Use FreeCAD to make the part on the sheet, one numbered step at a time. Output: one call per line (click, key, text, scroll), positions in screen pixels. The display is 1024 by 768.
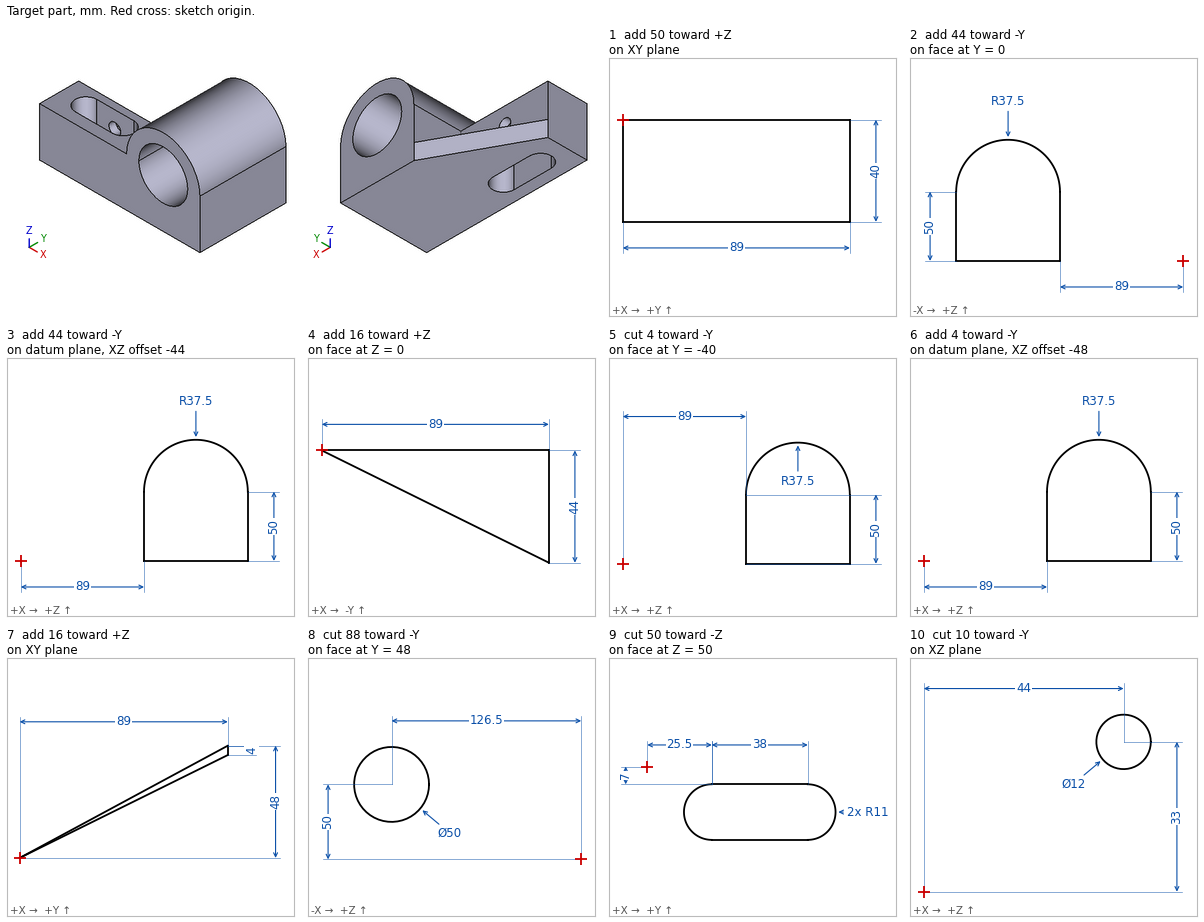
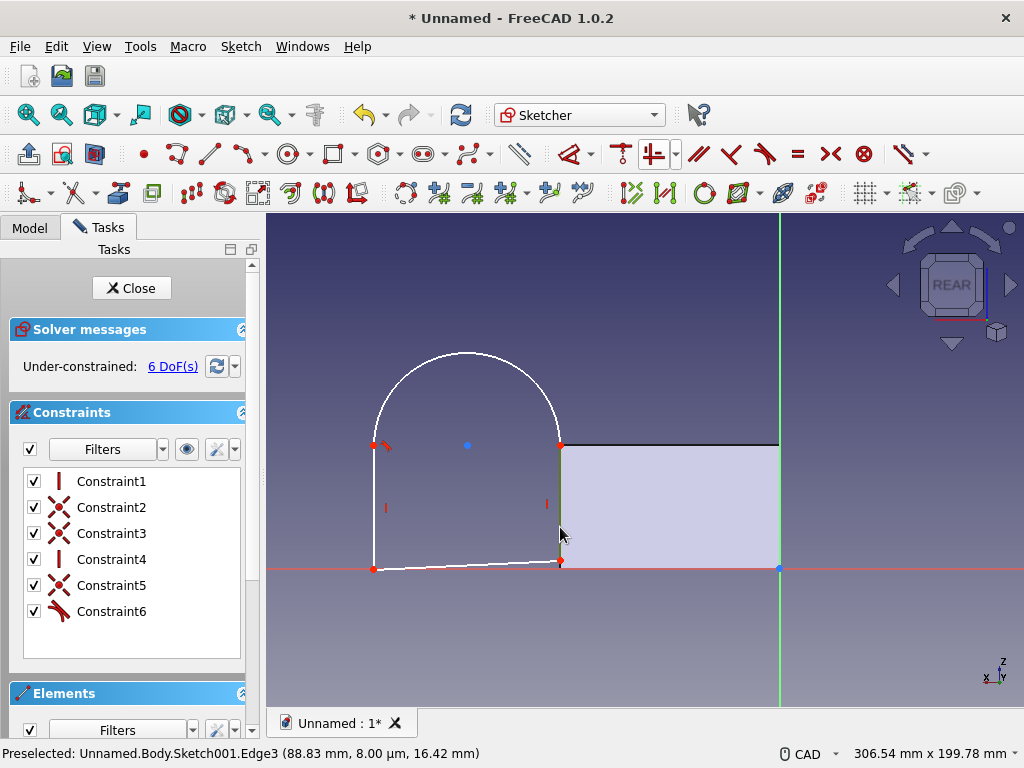
click(522, 371)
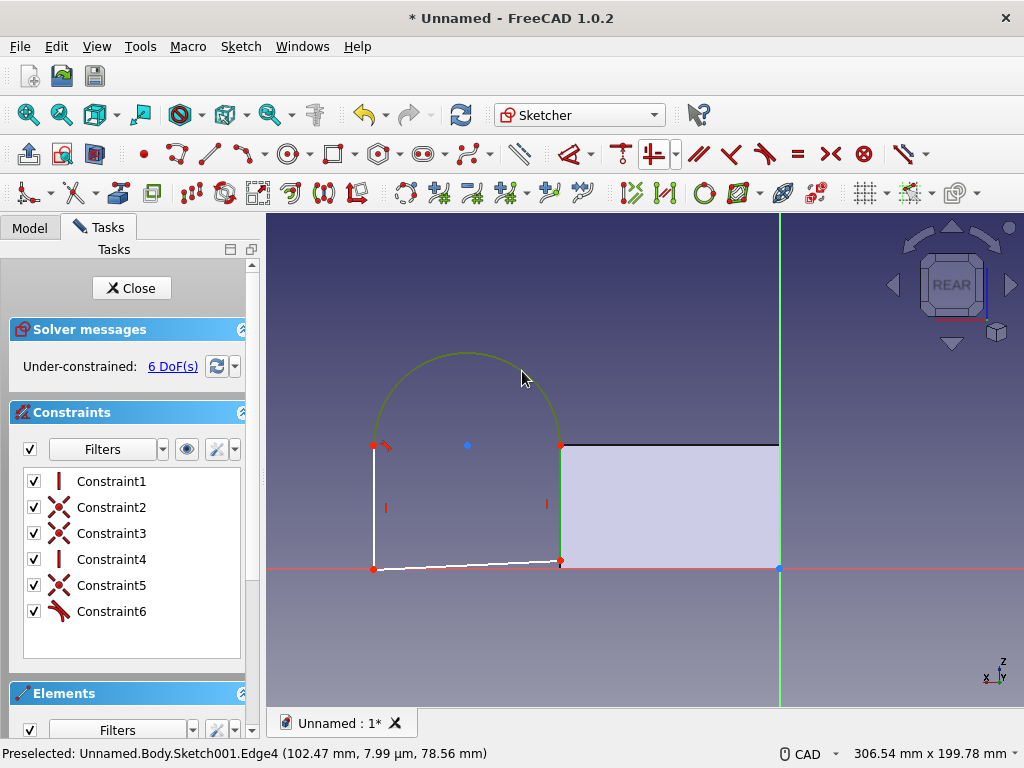
click(765, 154)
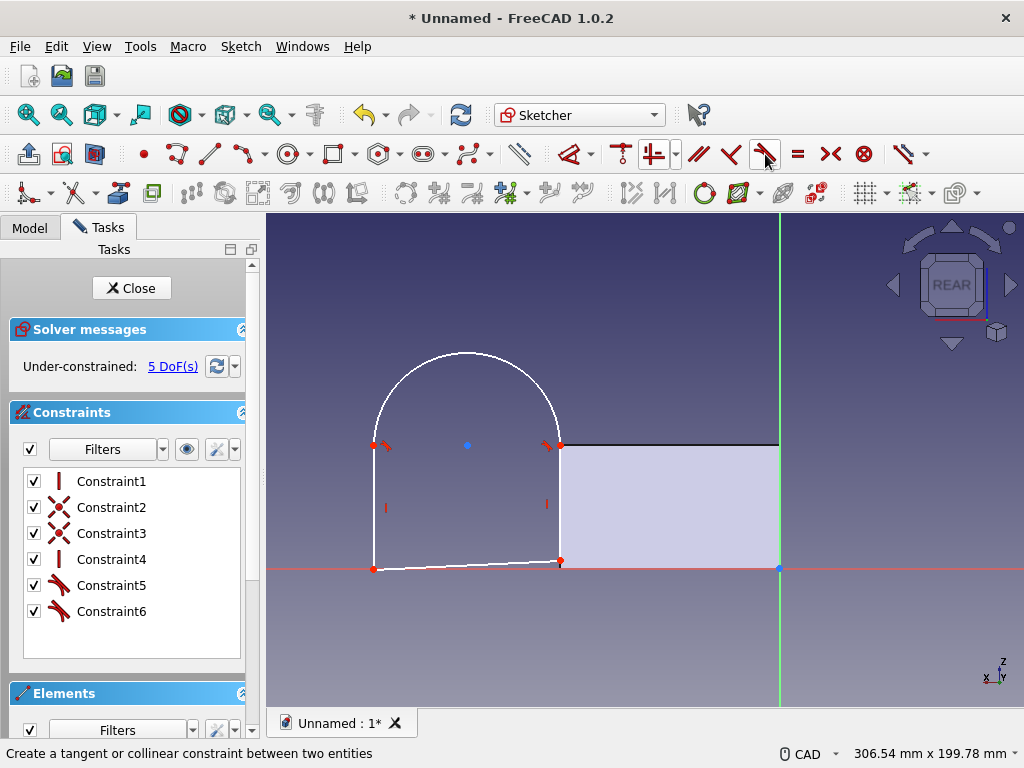
click(430, 567)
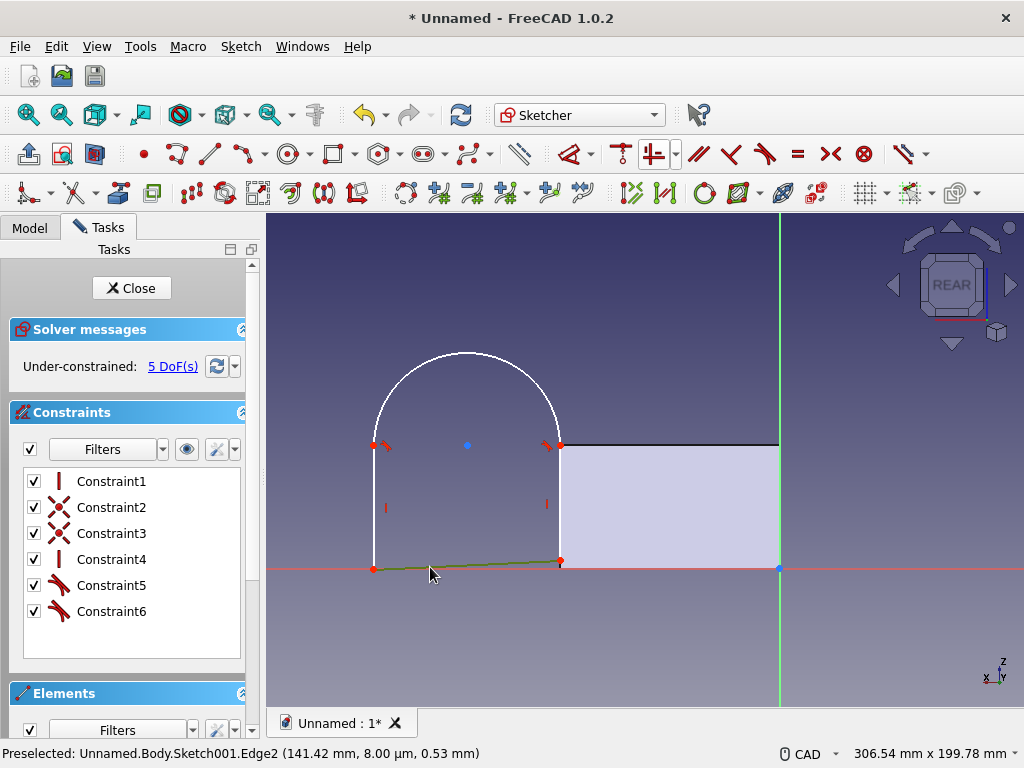
key(h)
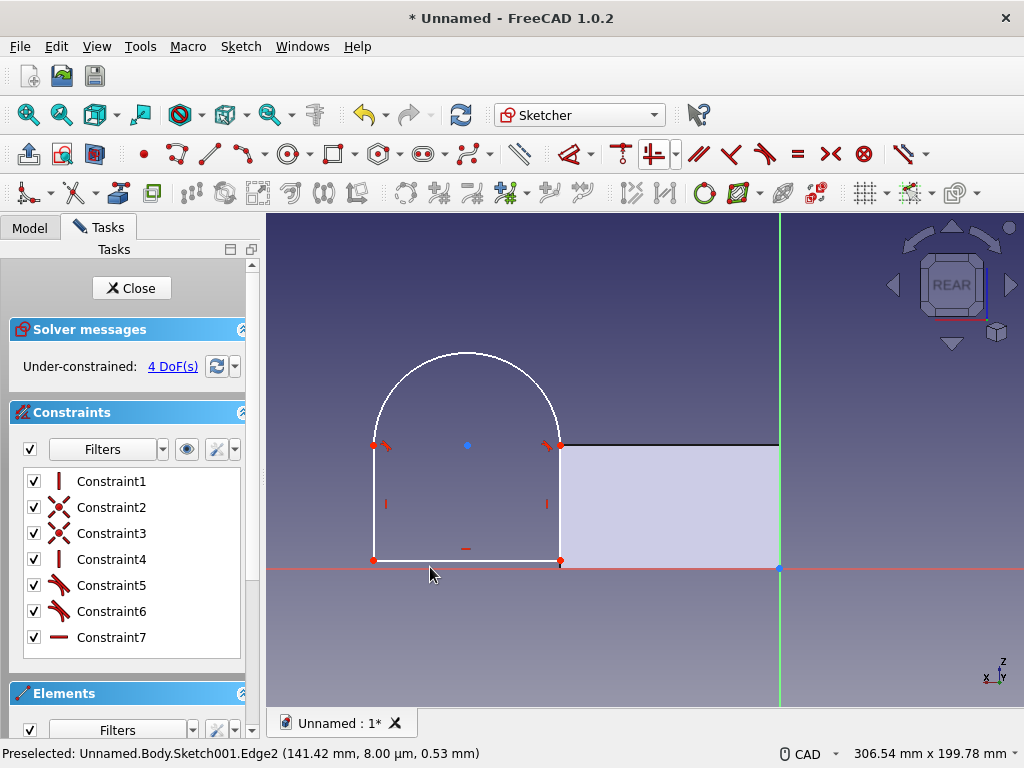
key(d)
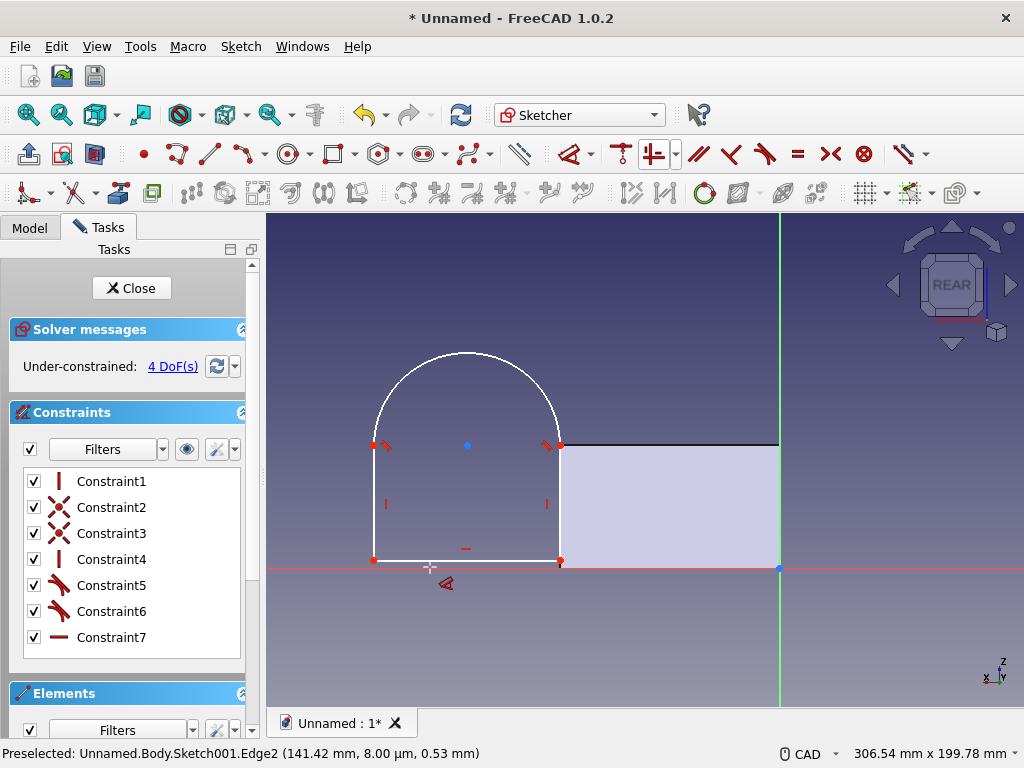
click(522, 371)
click(541, 345)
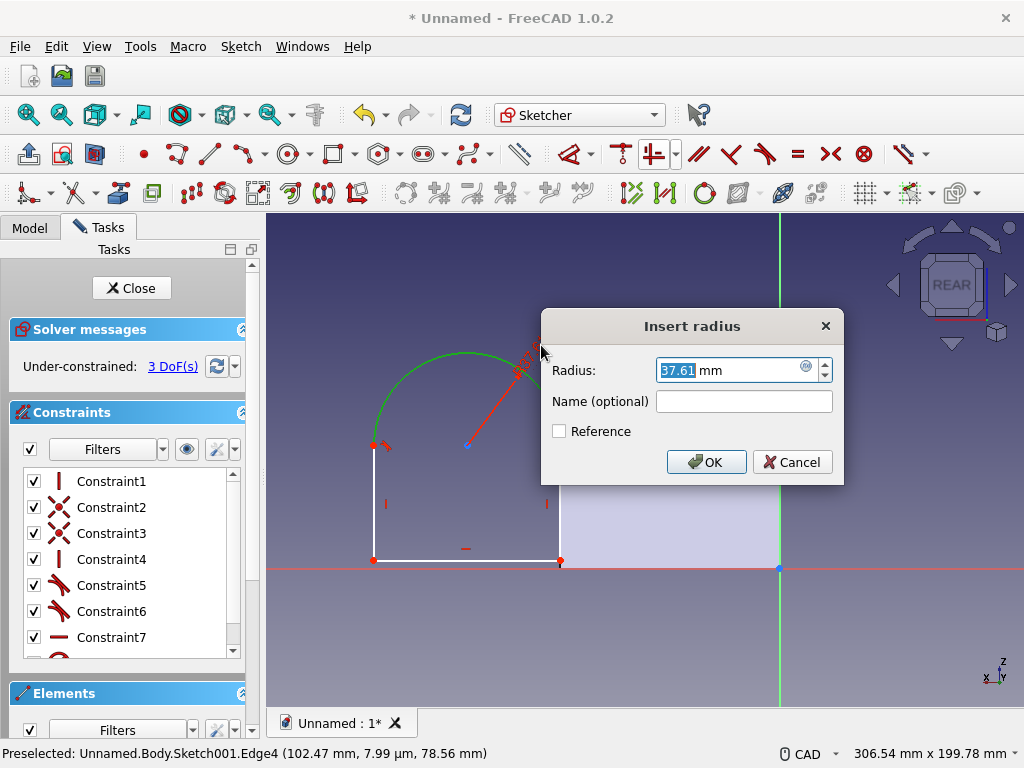
text(37.5)
key(Return)
key(Escape)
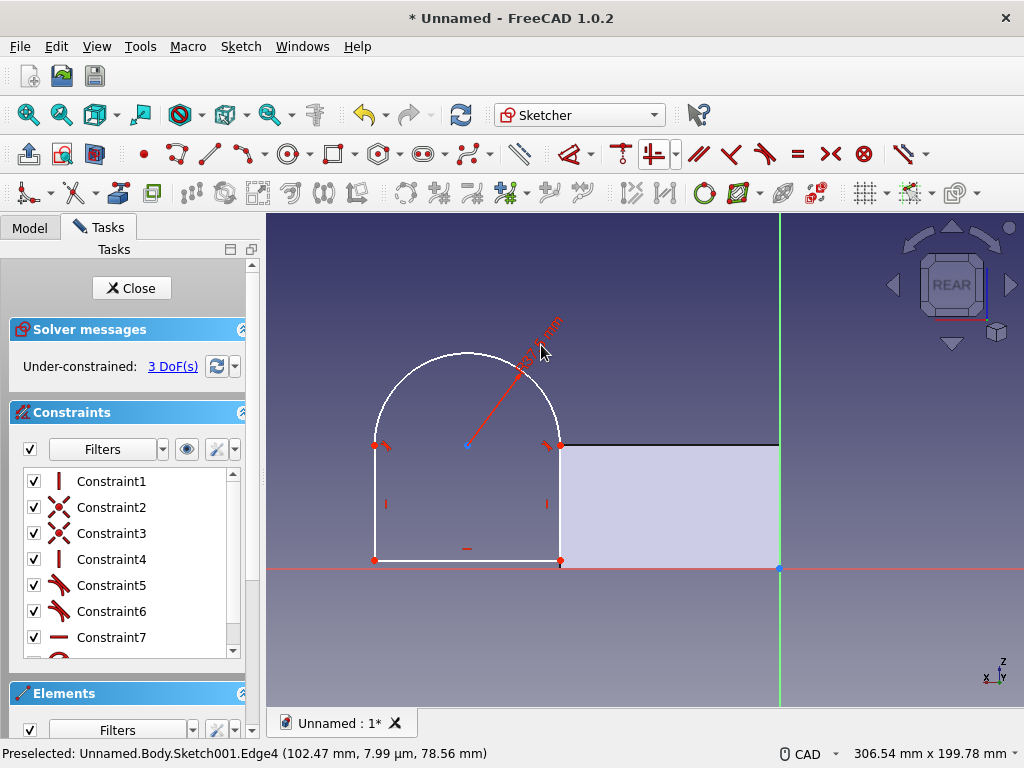
click(375, 561)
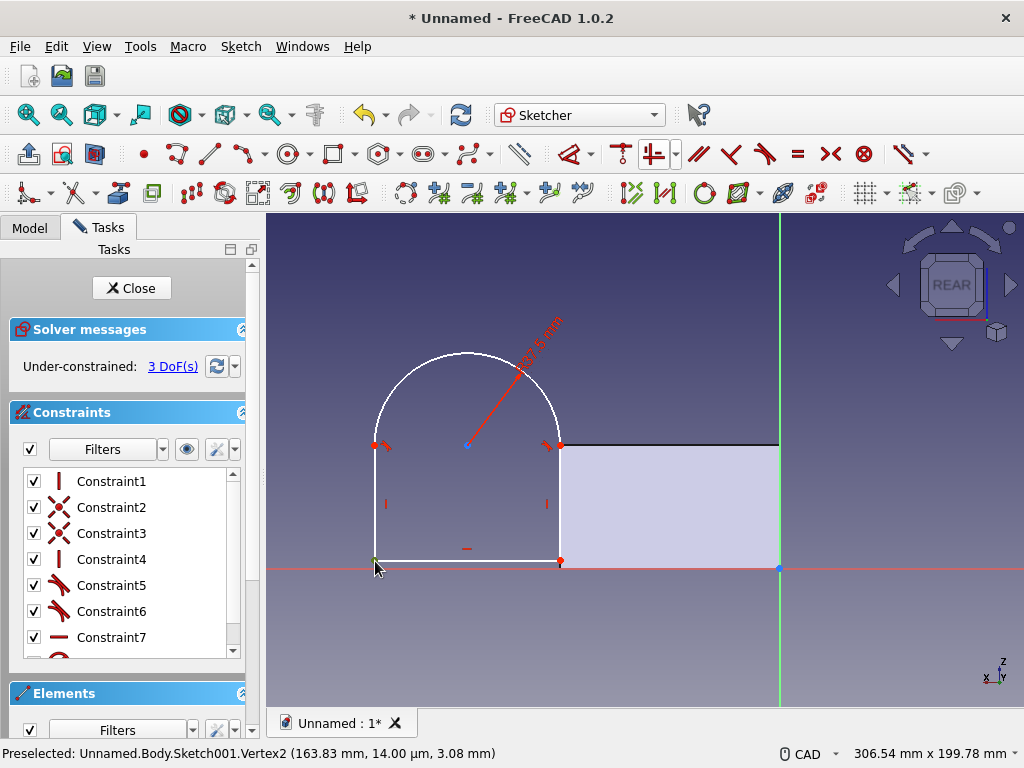
click(334, 569)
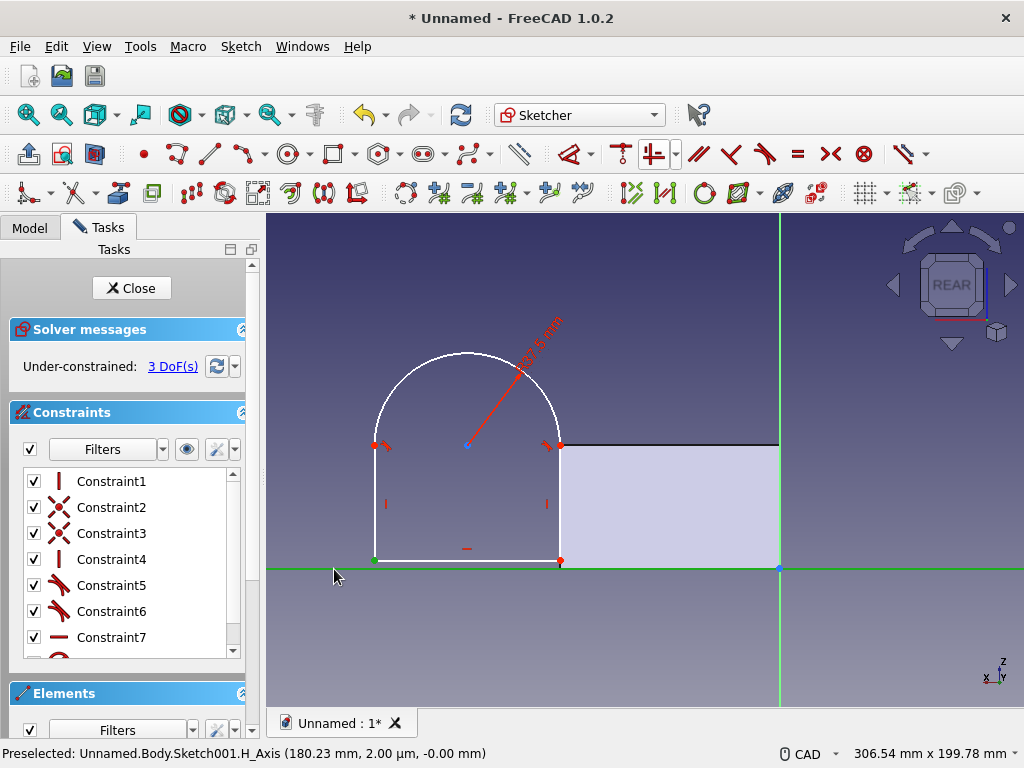
click(621, 154)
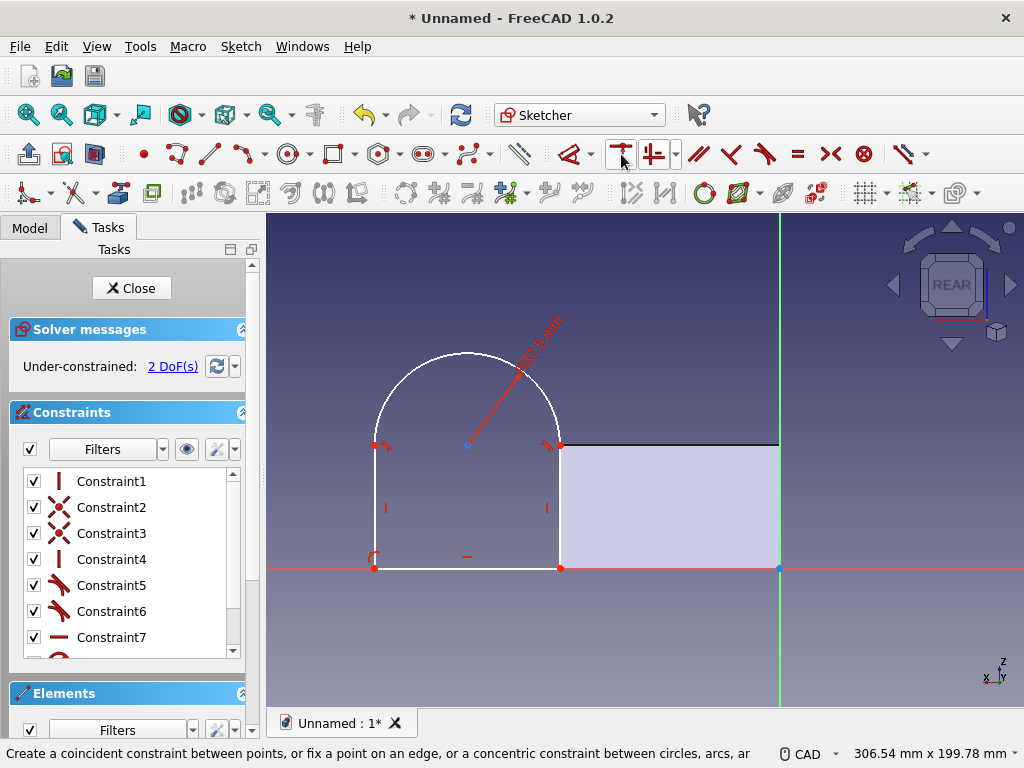
click(568, 154)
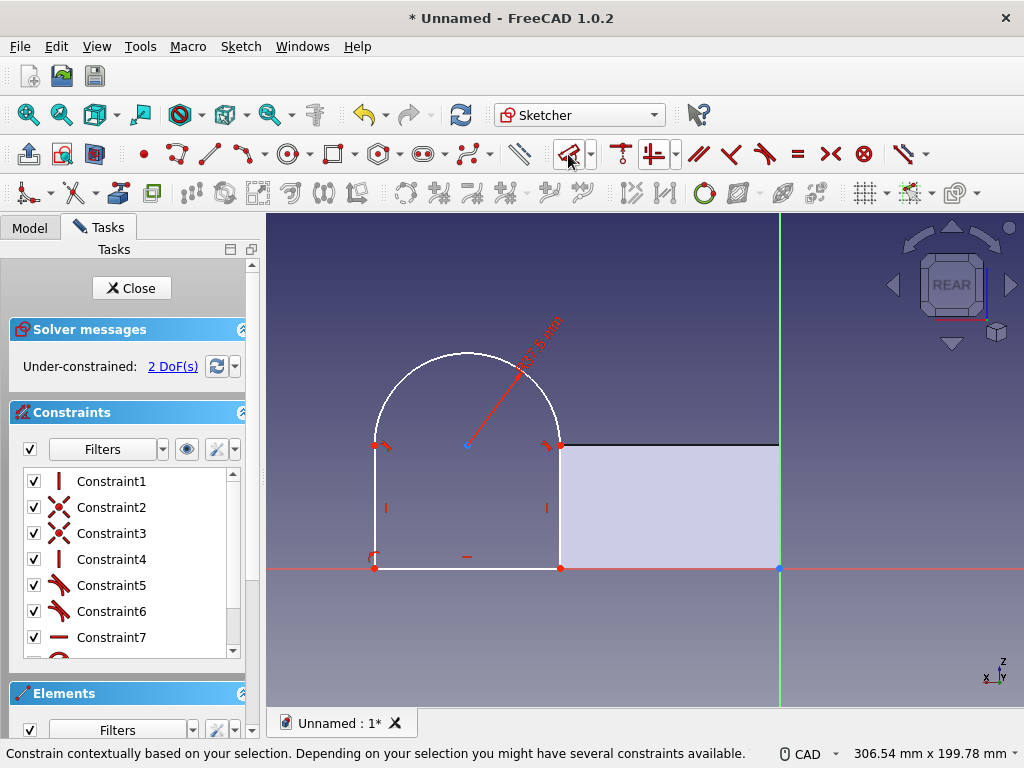
click(375, 483)
click(341, 507)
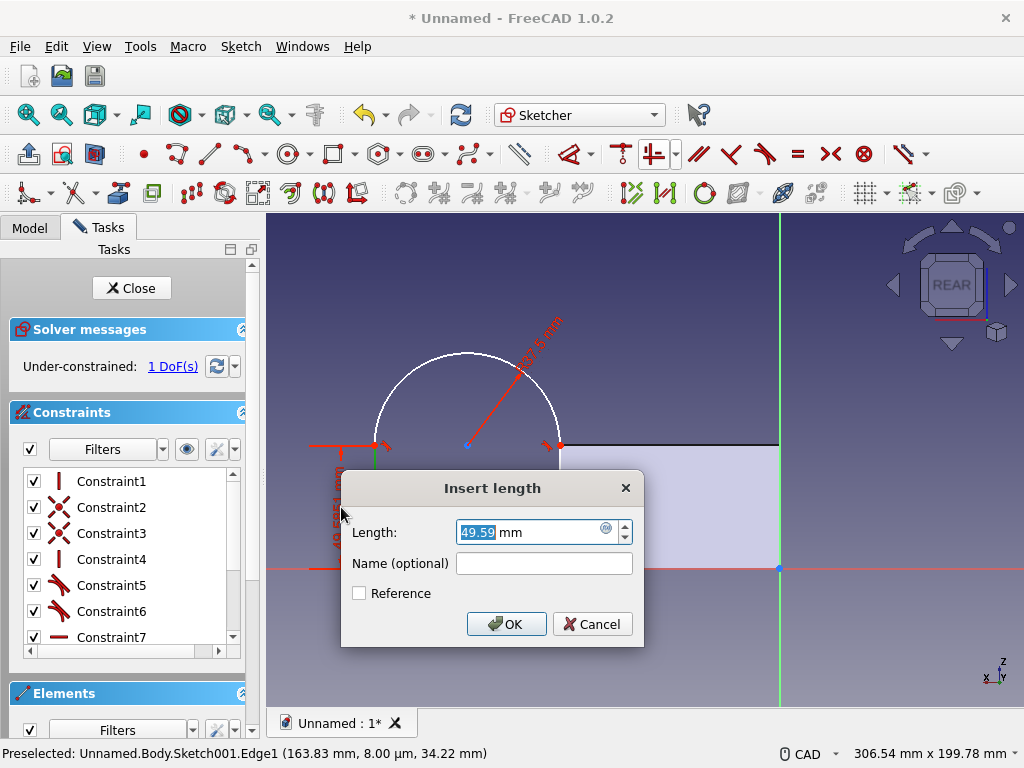
text(50)
key(Return)